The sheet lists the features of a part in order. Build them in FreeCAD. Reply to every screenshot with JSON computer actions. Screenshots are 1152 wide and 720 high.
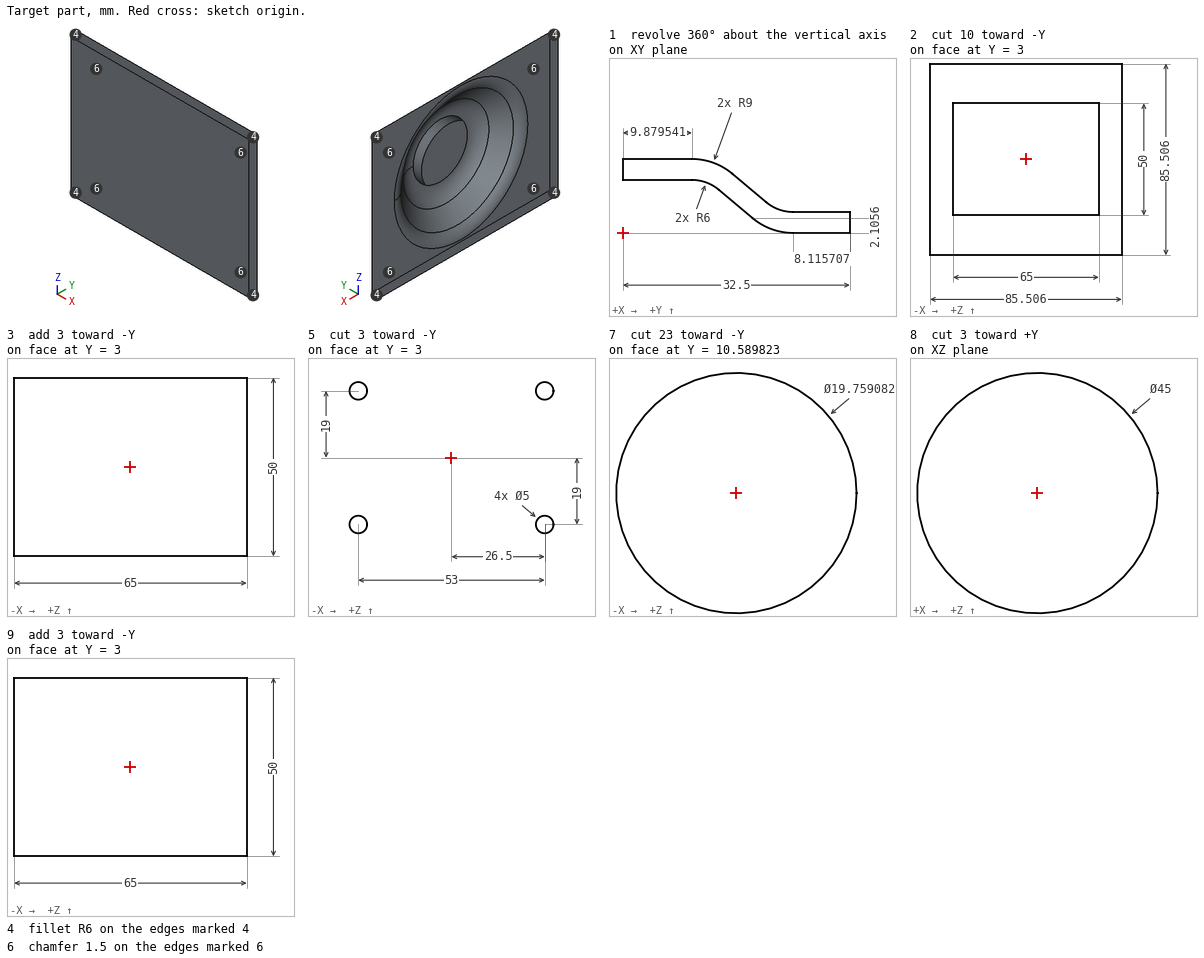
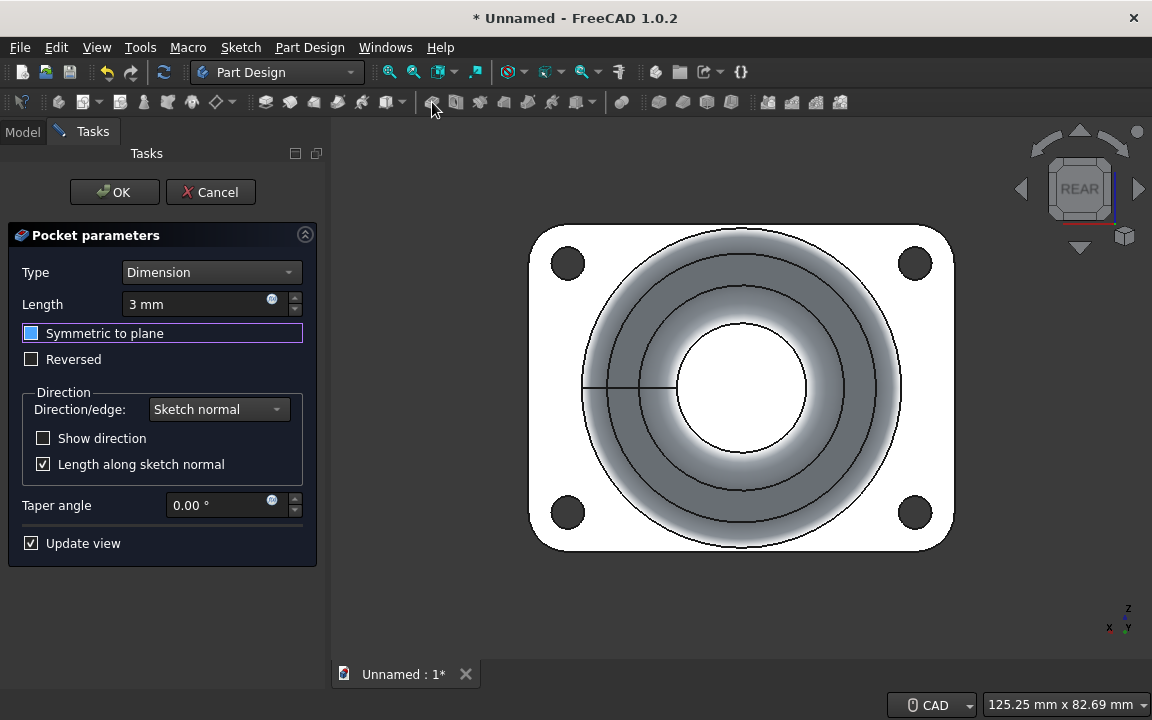
{"action": "left_click", "coordinate": [115, 192]}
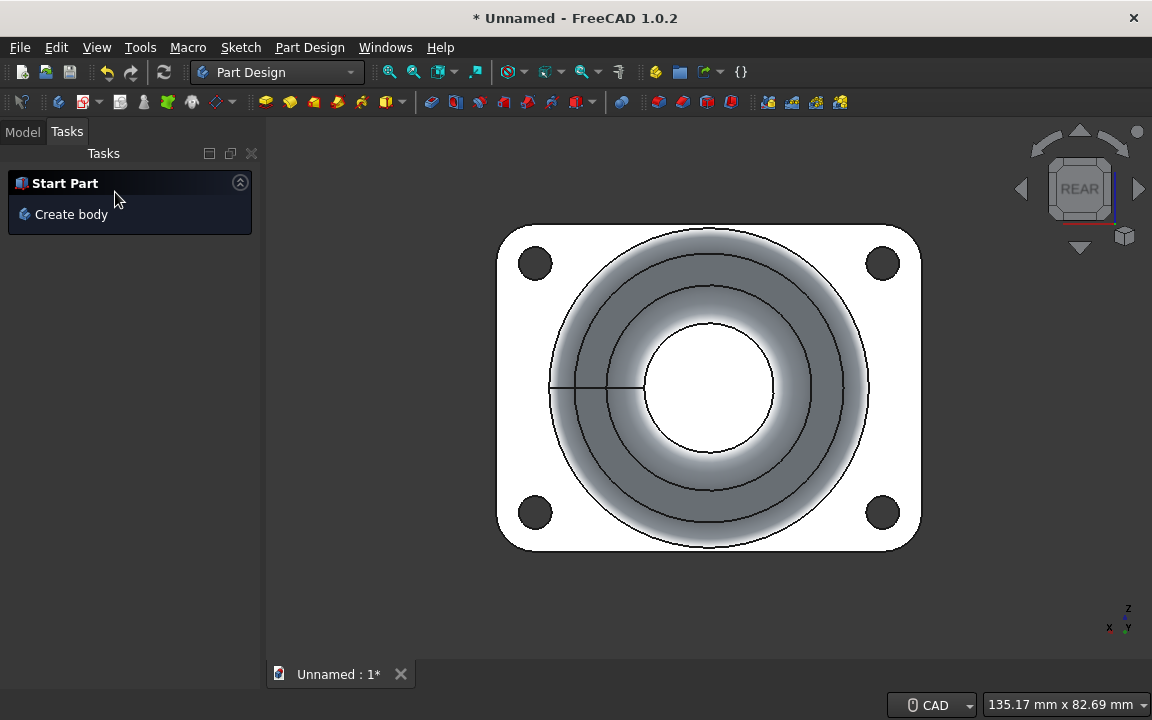
{"action": "left_click", "coordinate": [866, 262]}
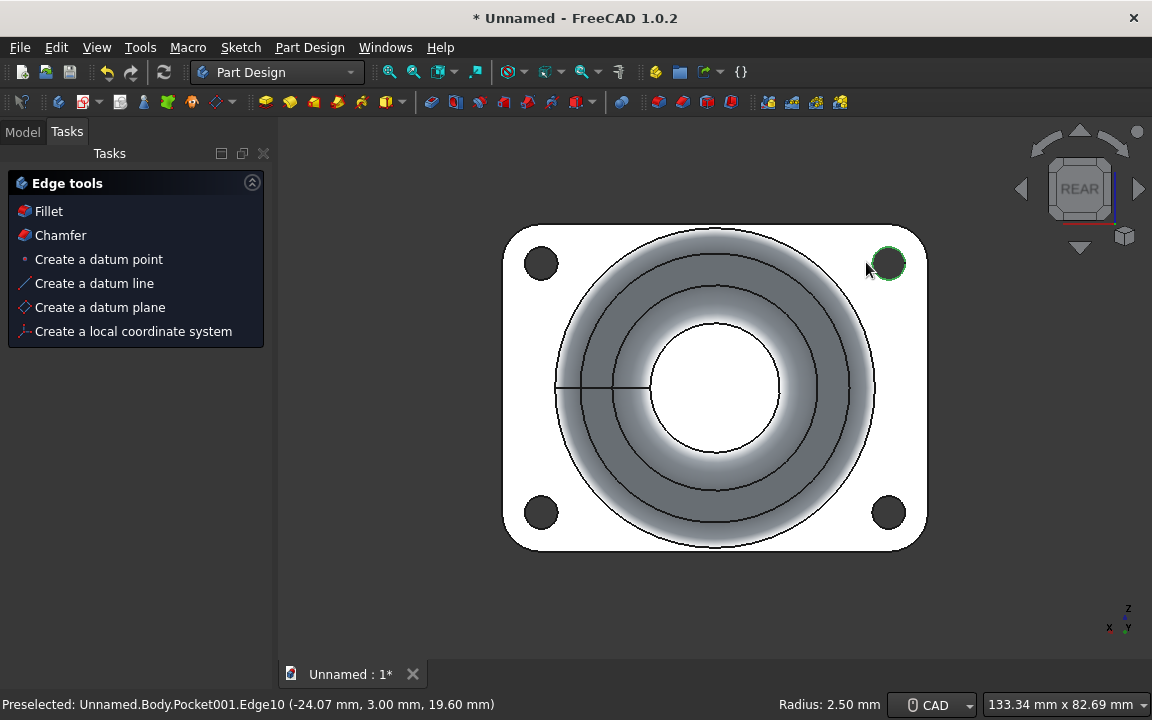
{"action": "left_click", "coordinate": [525, 262], "text": "ctrl"}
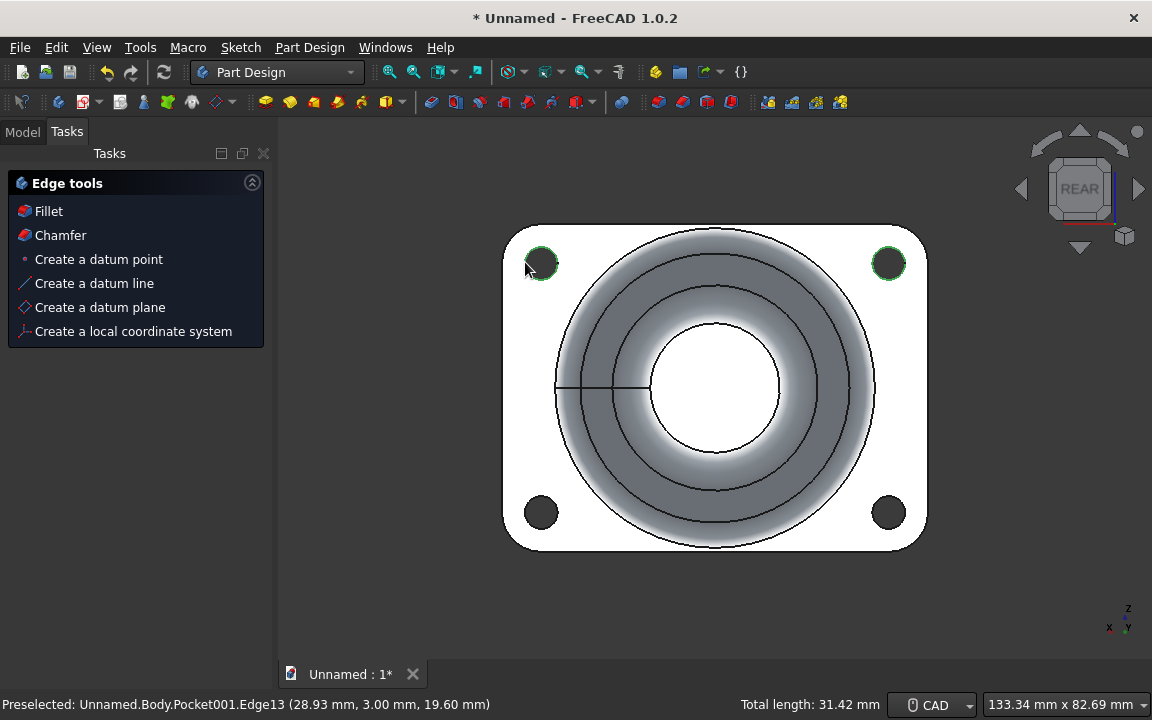
{"action": "left_click", "coordinate": [525, 512], "text": "ctrl"}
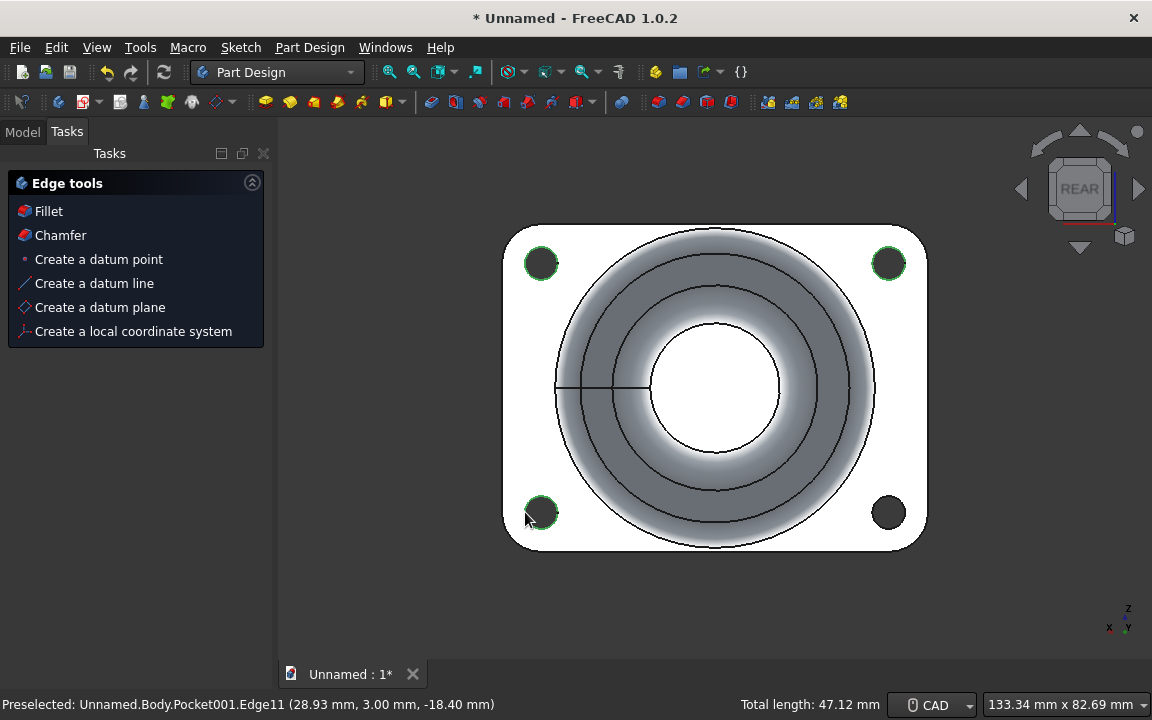
{"action": "left_click", "coordinate": [872, 512], "text": "ctrl"}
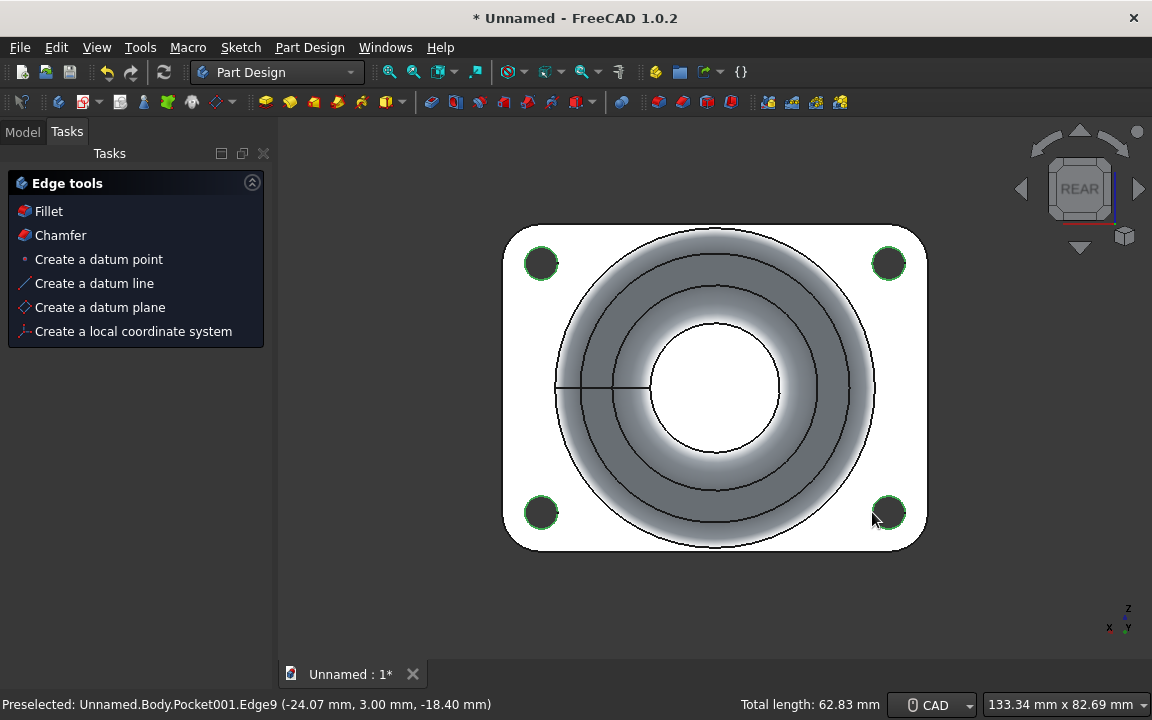
{"action": "left_click", "coordinate": [684, 102]}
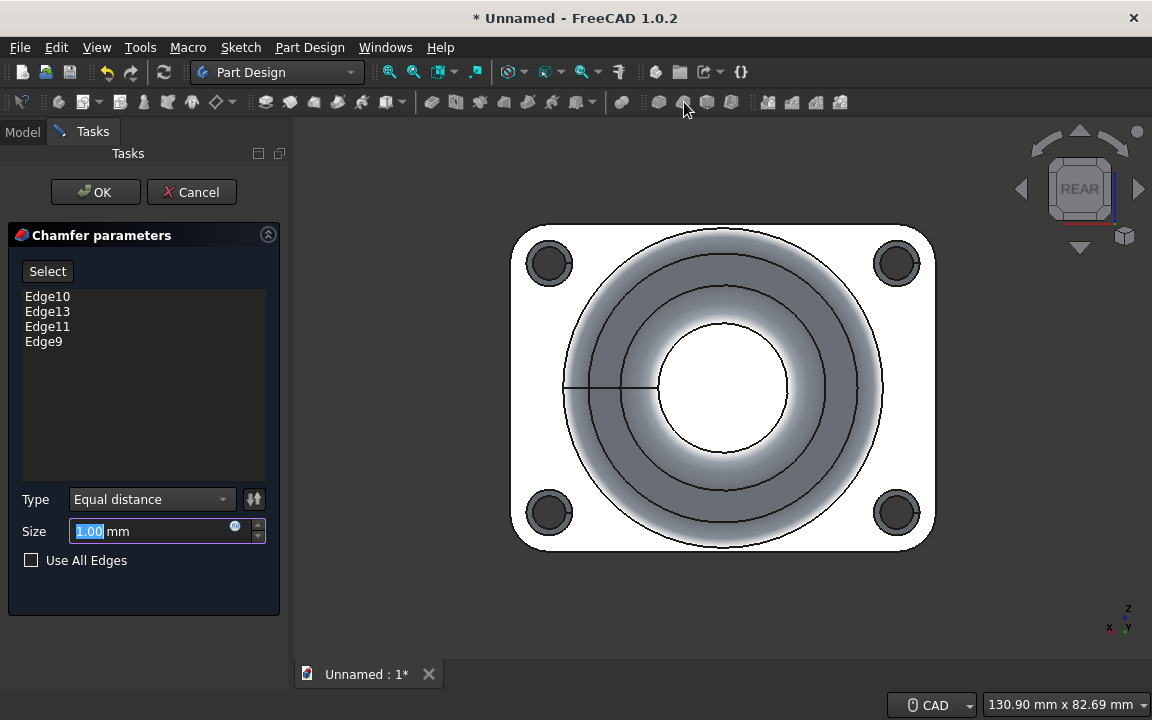
{"action": "type", "text": "1.5"}
{"action": "key", "text": "Tab"}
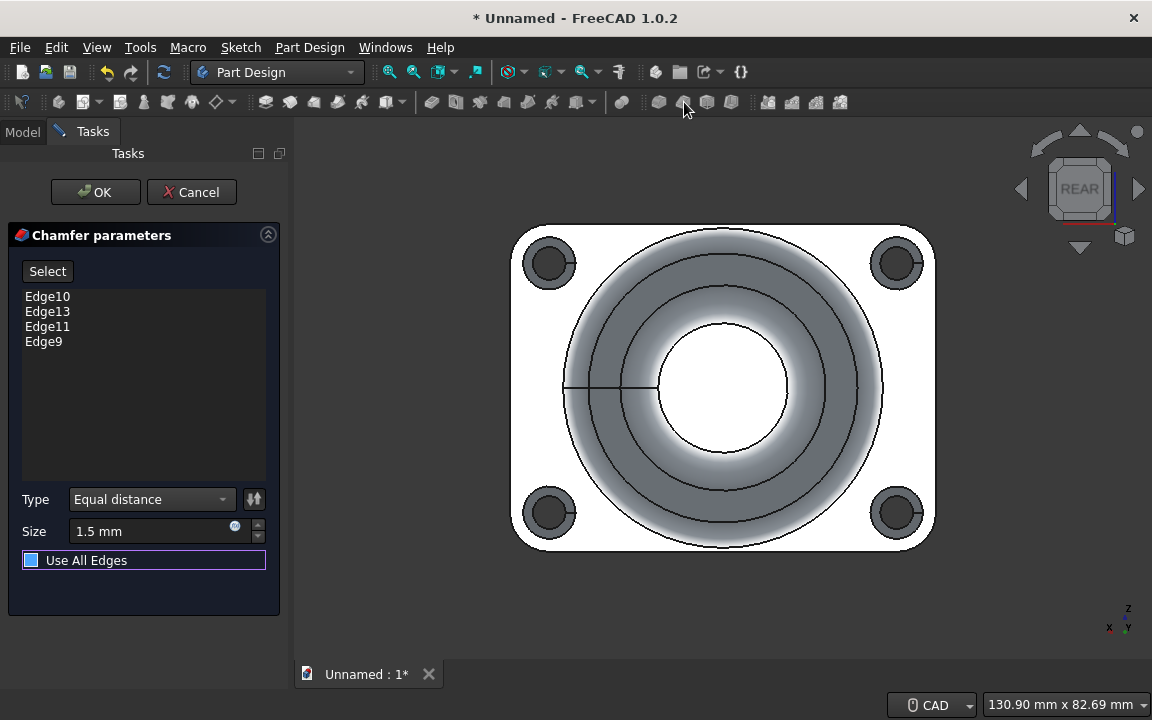
{"action": "left_click", "coordinate": [96, 192]}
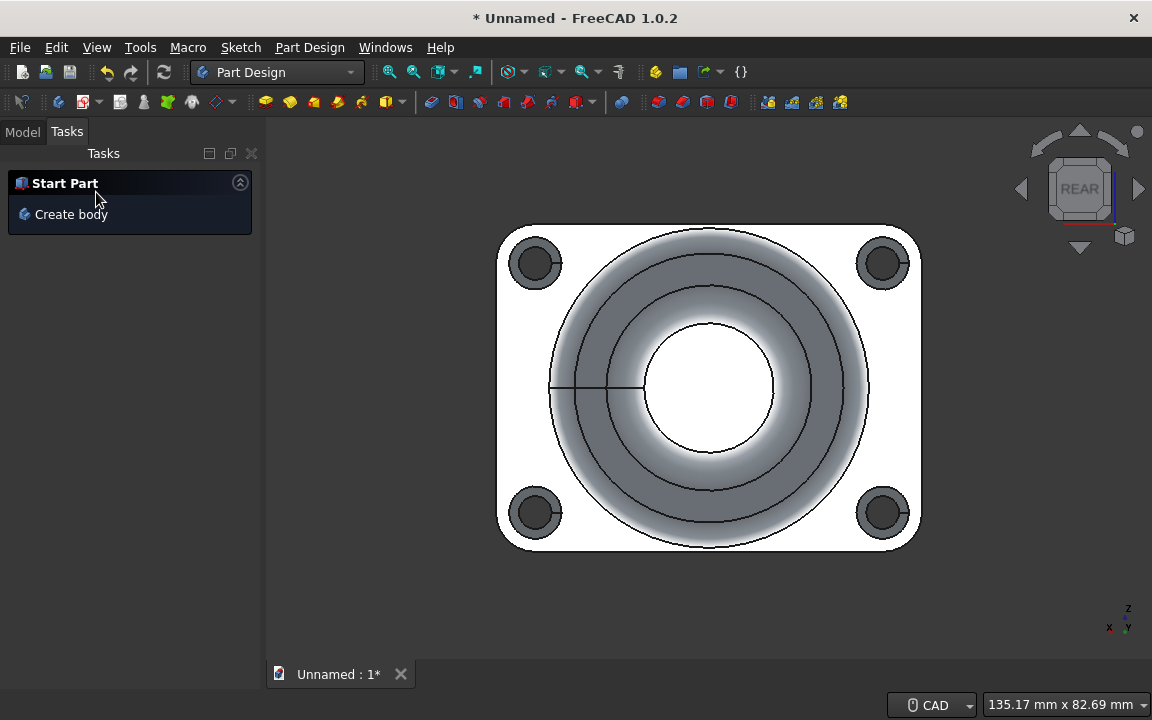
{"action": "left_click", "coordinate": [709, 387]}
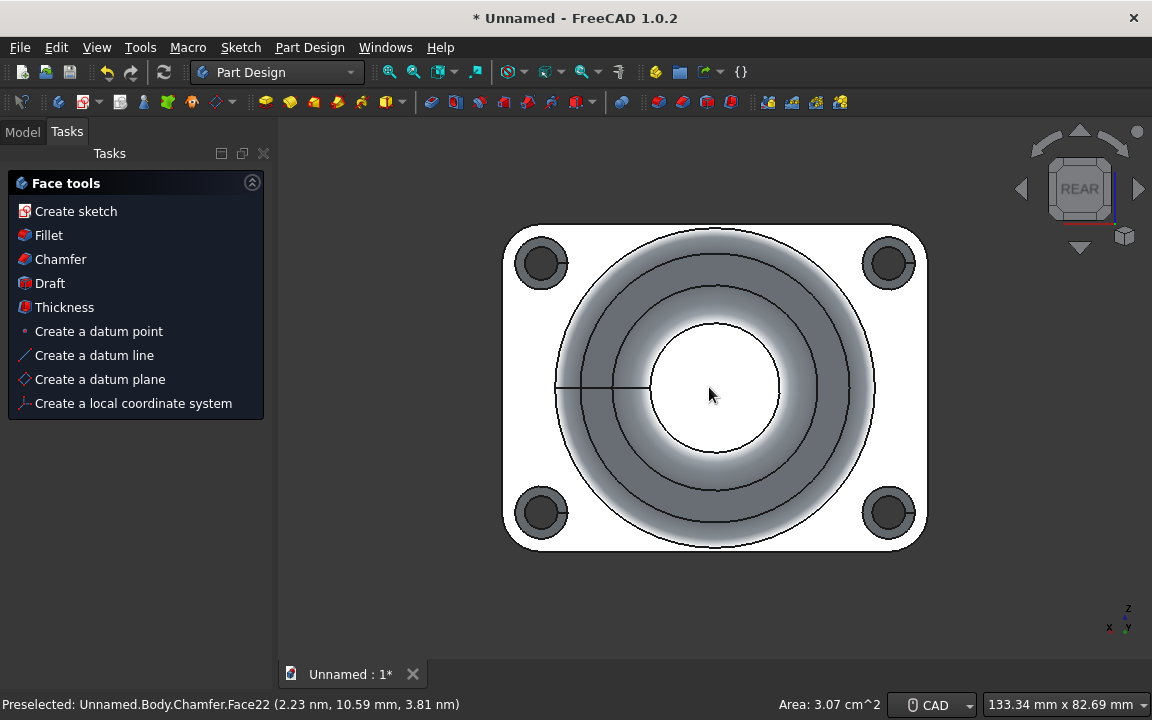
{"action": "left_click", "coordinate": [84, 102]}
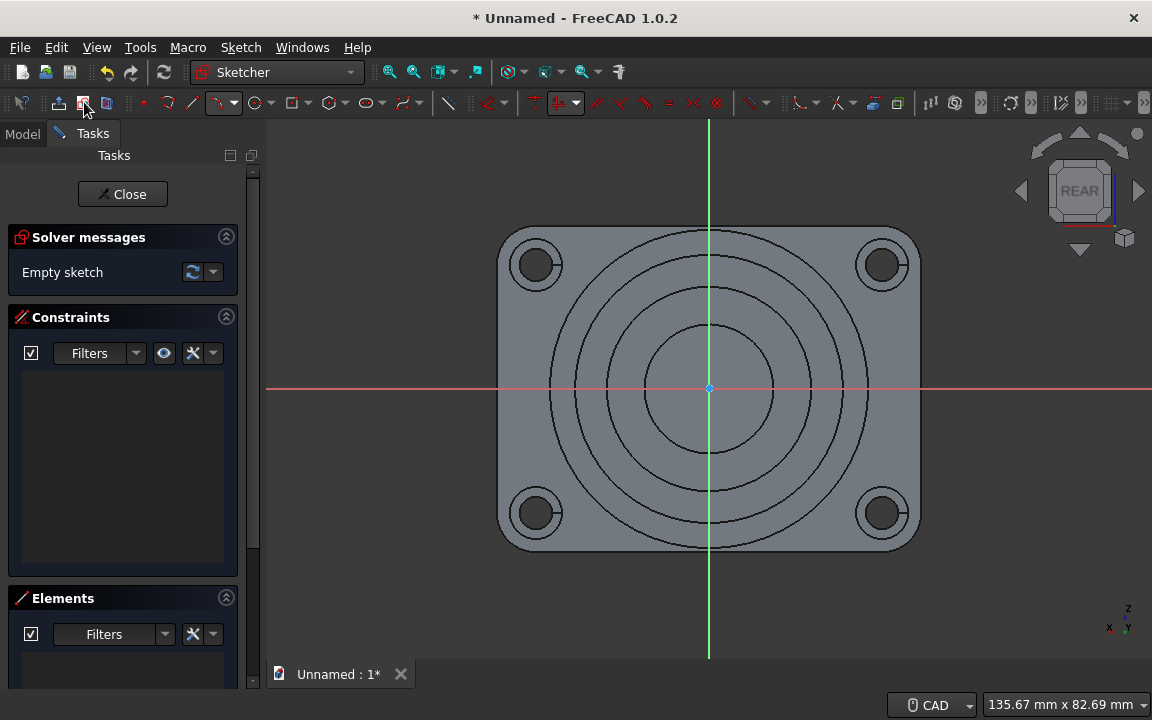
{"action": "scroll", "coordinate": [749, 389], "scroll_direction": "up", "scroll_amount": 5}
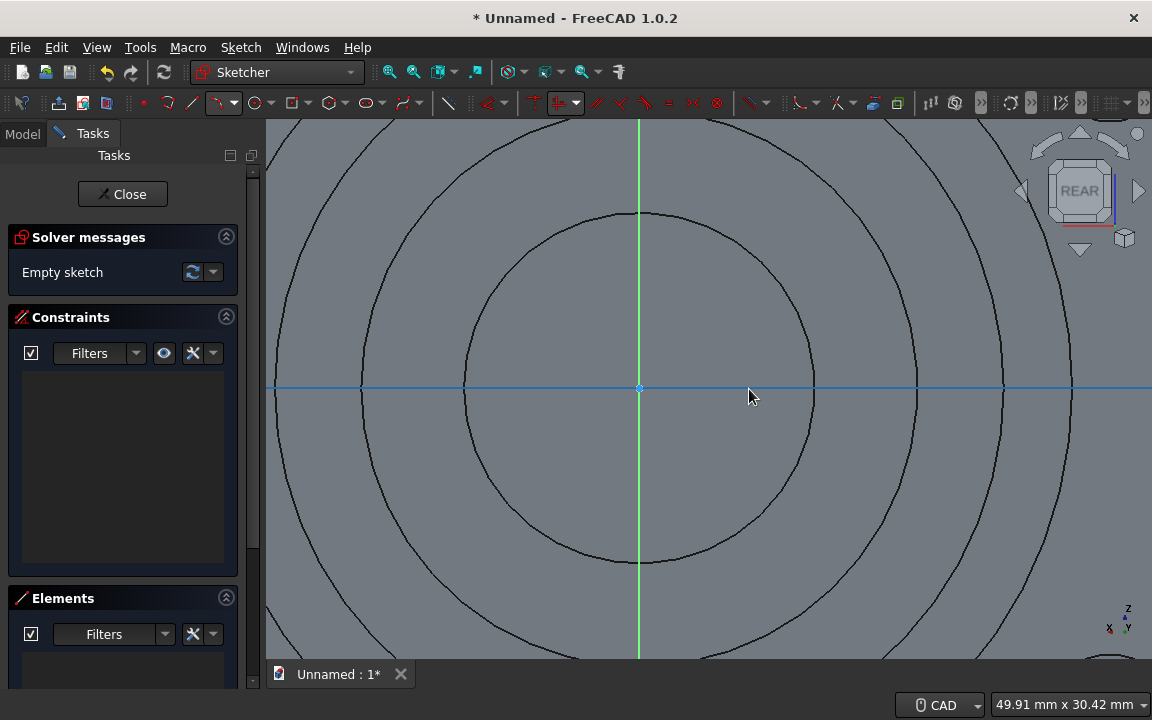
{"action": "left_click", "coordinate": [256, 104]}